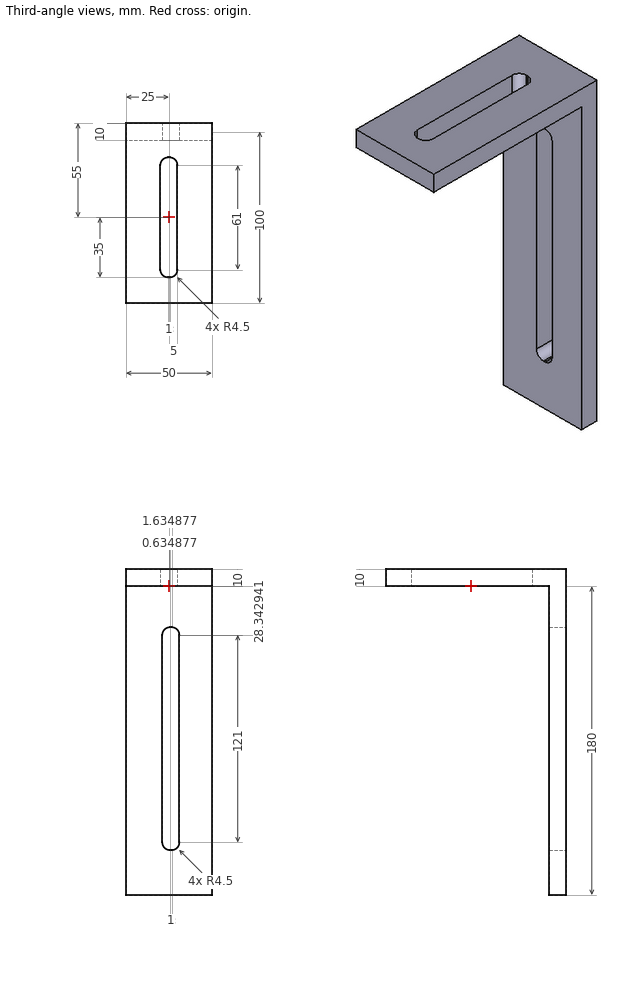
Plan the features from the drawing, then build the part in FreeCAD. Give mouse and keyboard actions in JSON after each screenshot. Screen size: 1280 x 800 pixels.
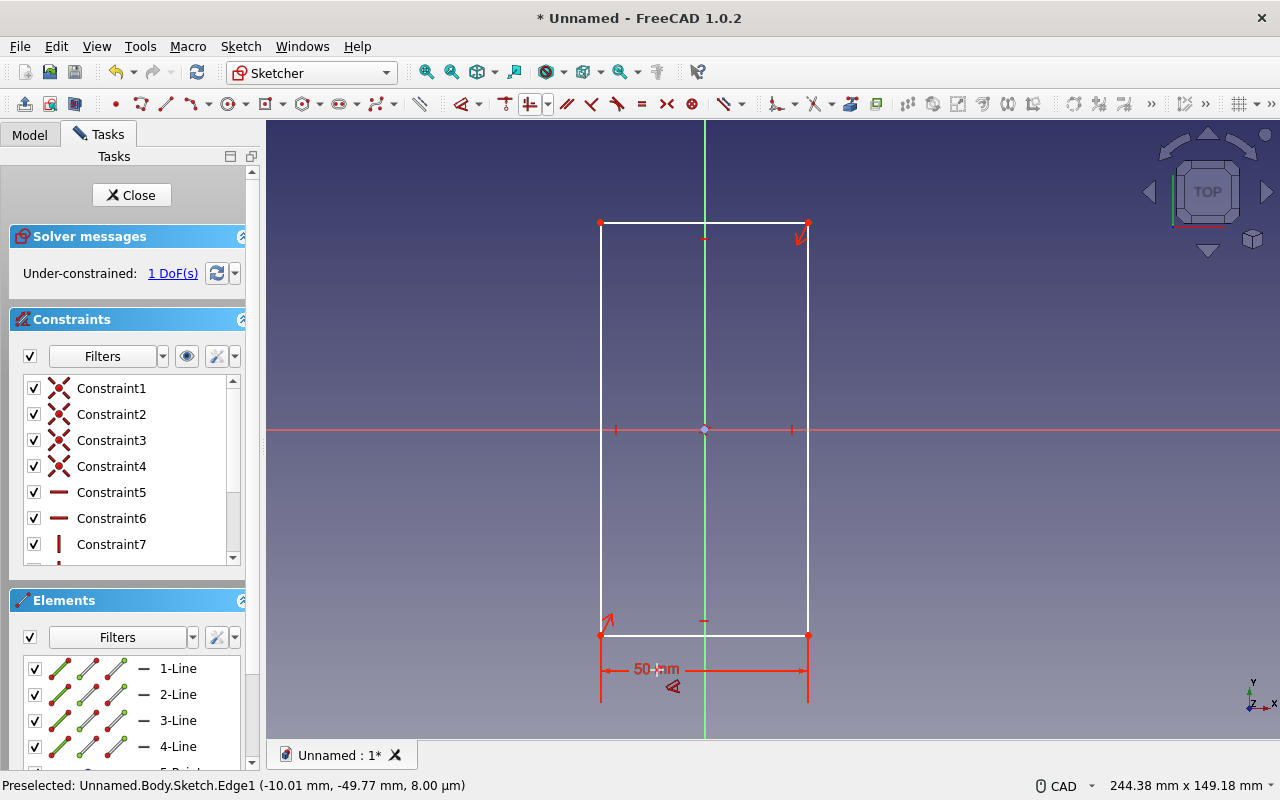
{"action": "left_click", "coordinate": [808, 512]}
{"action": "left_click", "coordinate": [842, 335]}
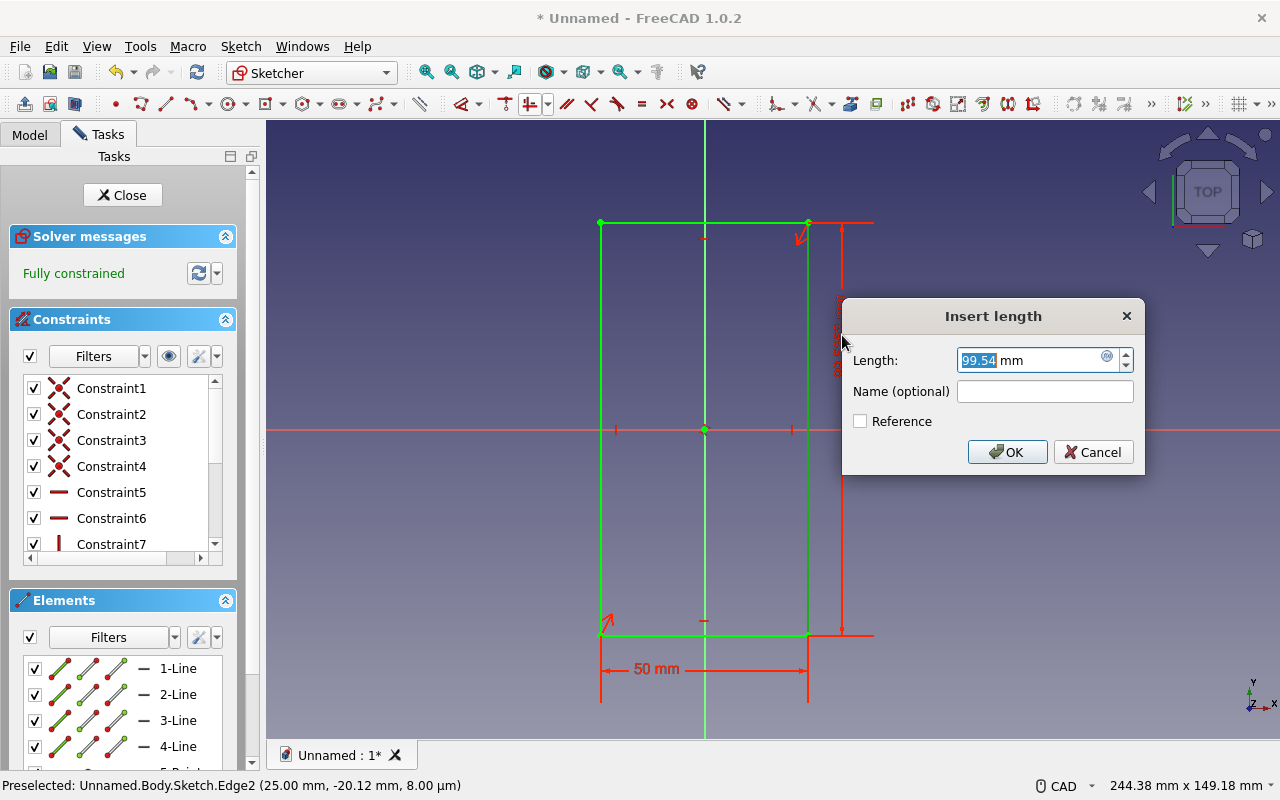
{"action": "type", "text": "100"}
{"action": "key", "text": "Return"}
{"action": "key", "text": "Escape"}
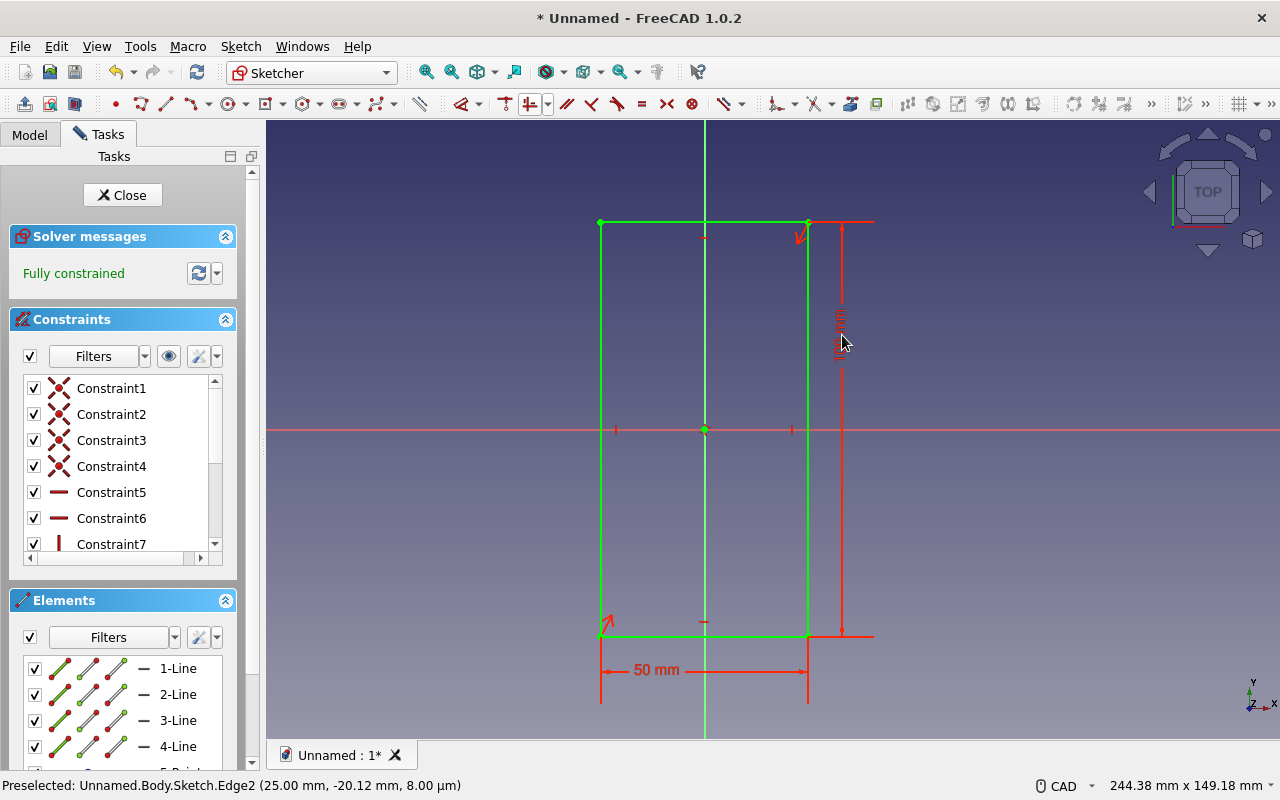
{"action": "left_click", "coordinate": [123, 195]}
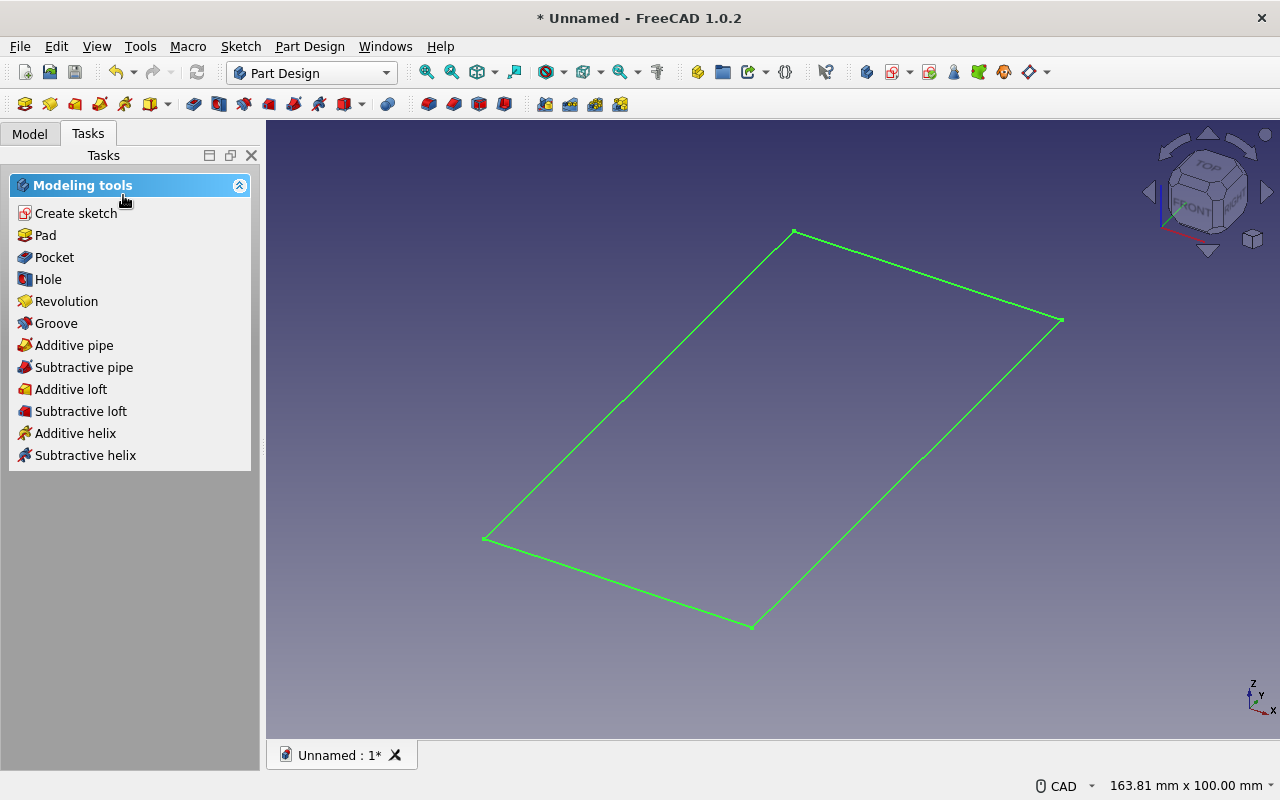
{"action": "left_click", "coordinate": [25, 104]}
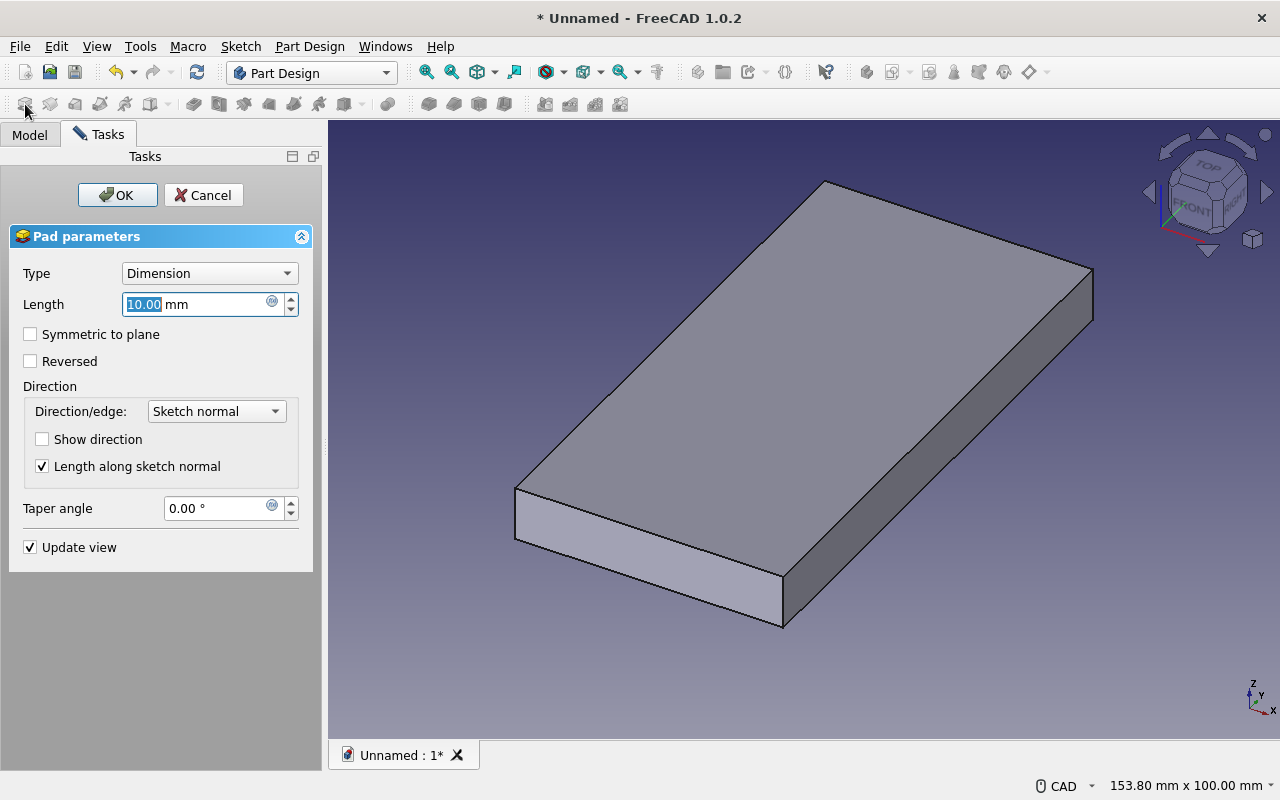
{"action": "type", "text": "10"}
{"action": "key", "text": "Tab"}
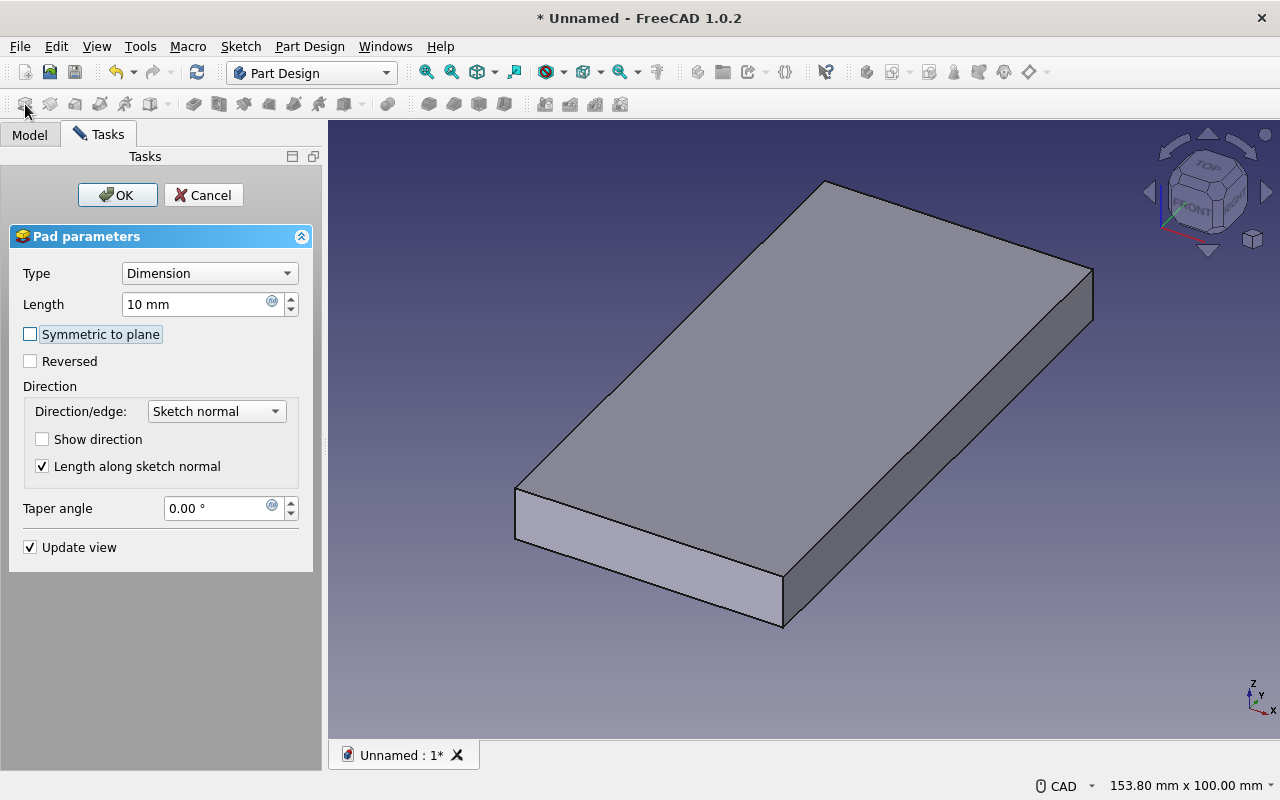
{"action": "left_click", "coordinate": [118, 195]}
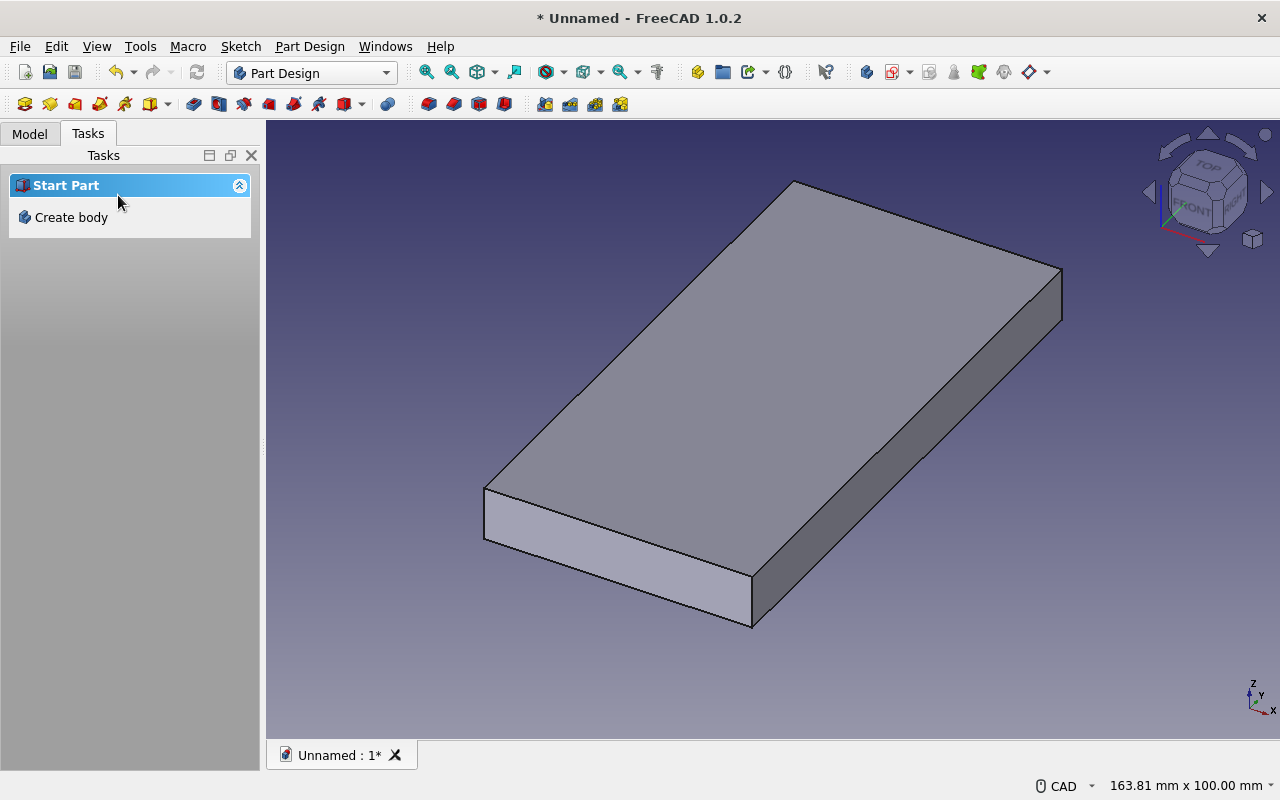
{"action": "left_click", "coordinate": [817, 334]}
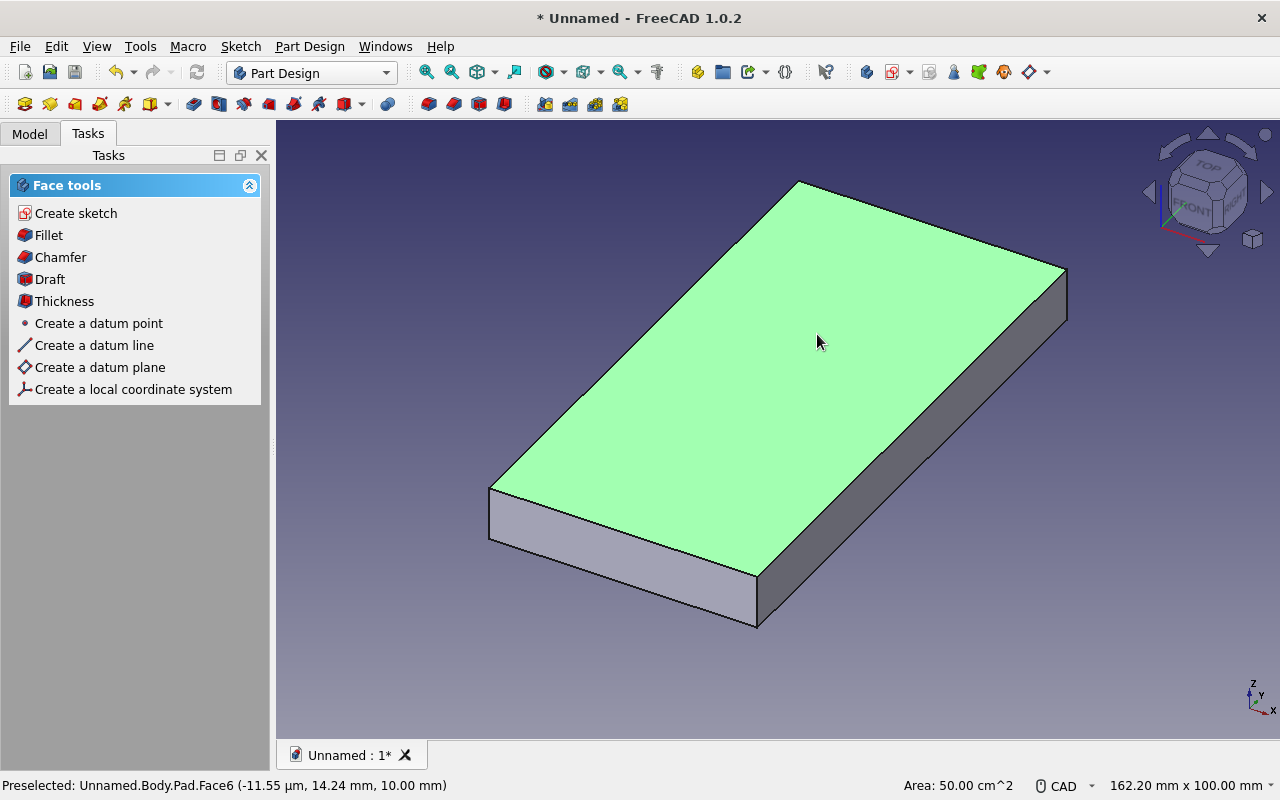
{"action": "left_click", "coordinate": [892, 72]}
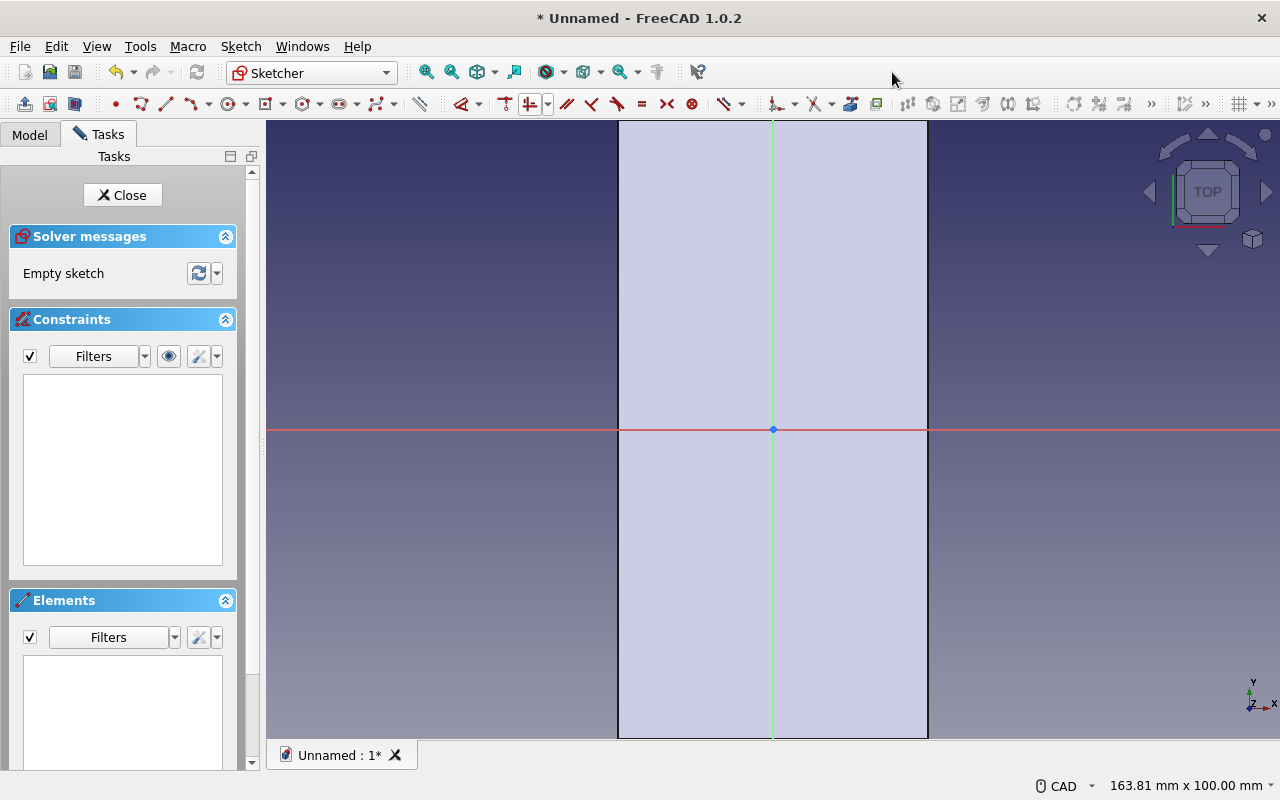
{"action": "left_click", "coordinate": [166, 104]}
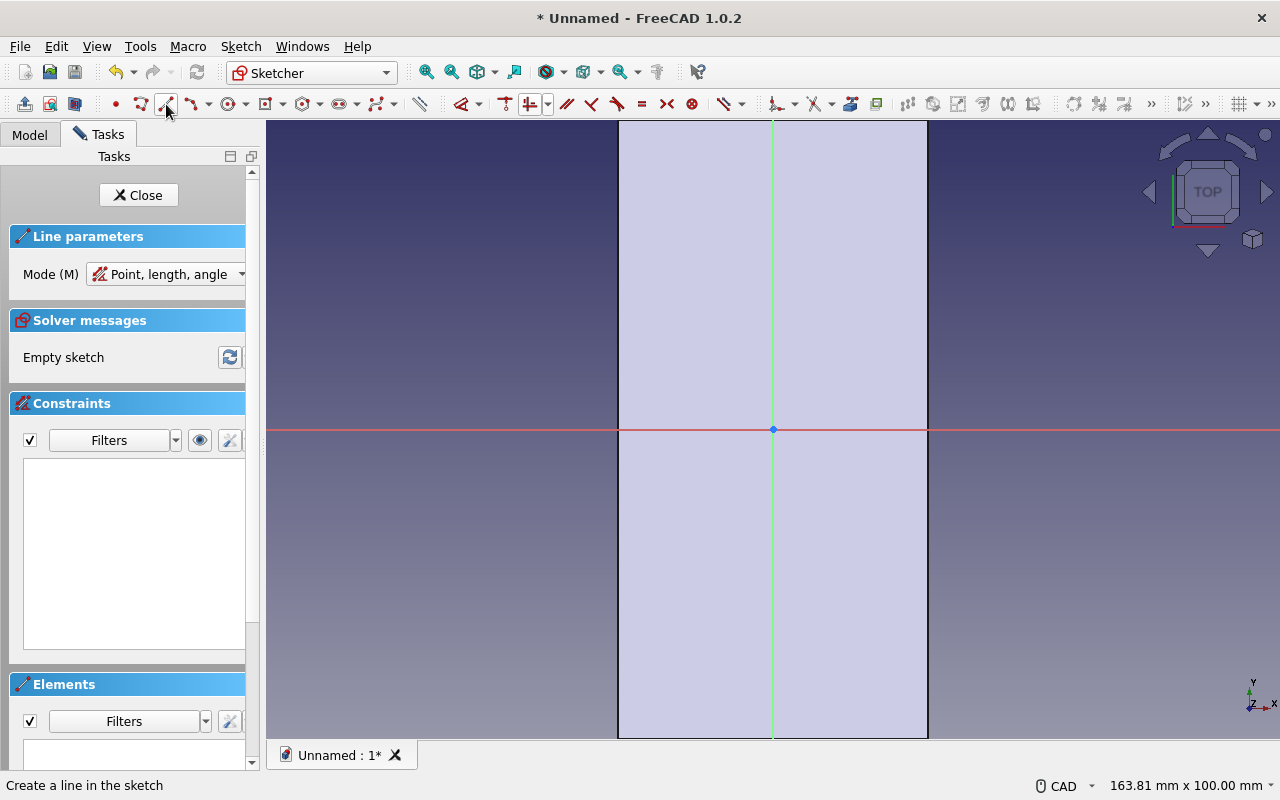
{"action": "scroll", "coordinate": [770, 646], "scroll_direction": "up", "scroll_amount": 9}